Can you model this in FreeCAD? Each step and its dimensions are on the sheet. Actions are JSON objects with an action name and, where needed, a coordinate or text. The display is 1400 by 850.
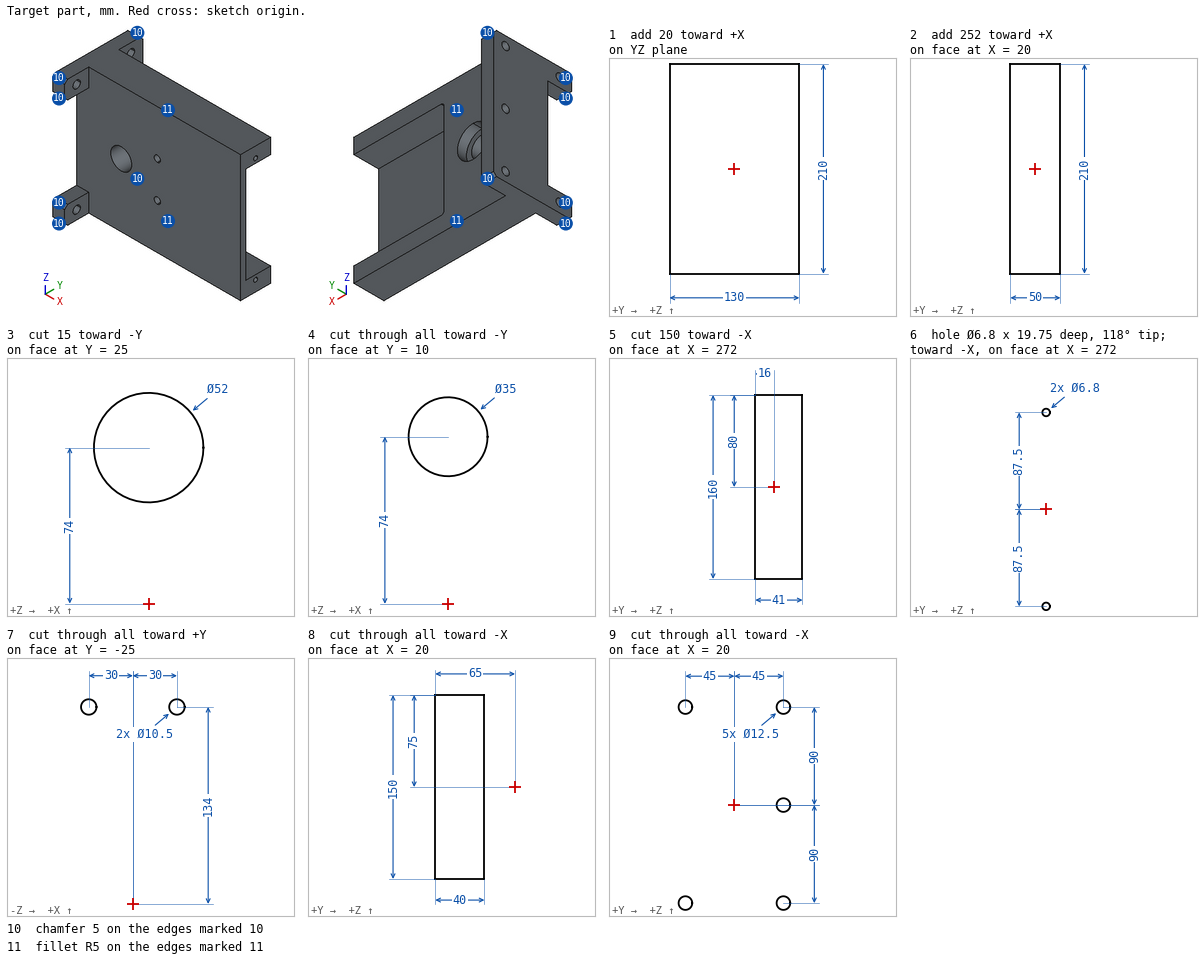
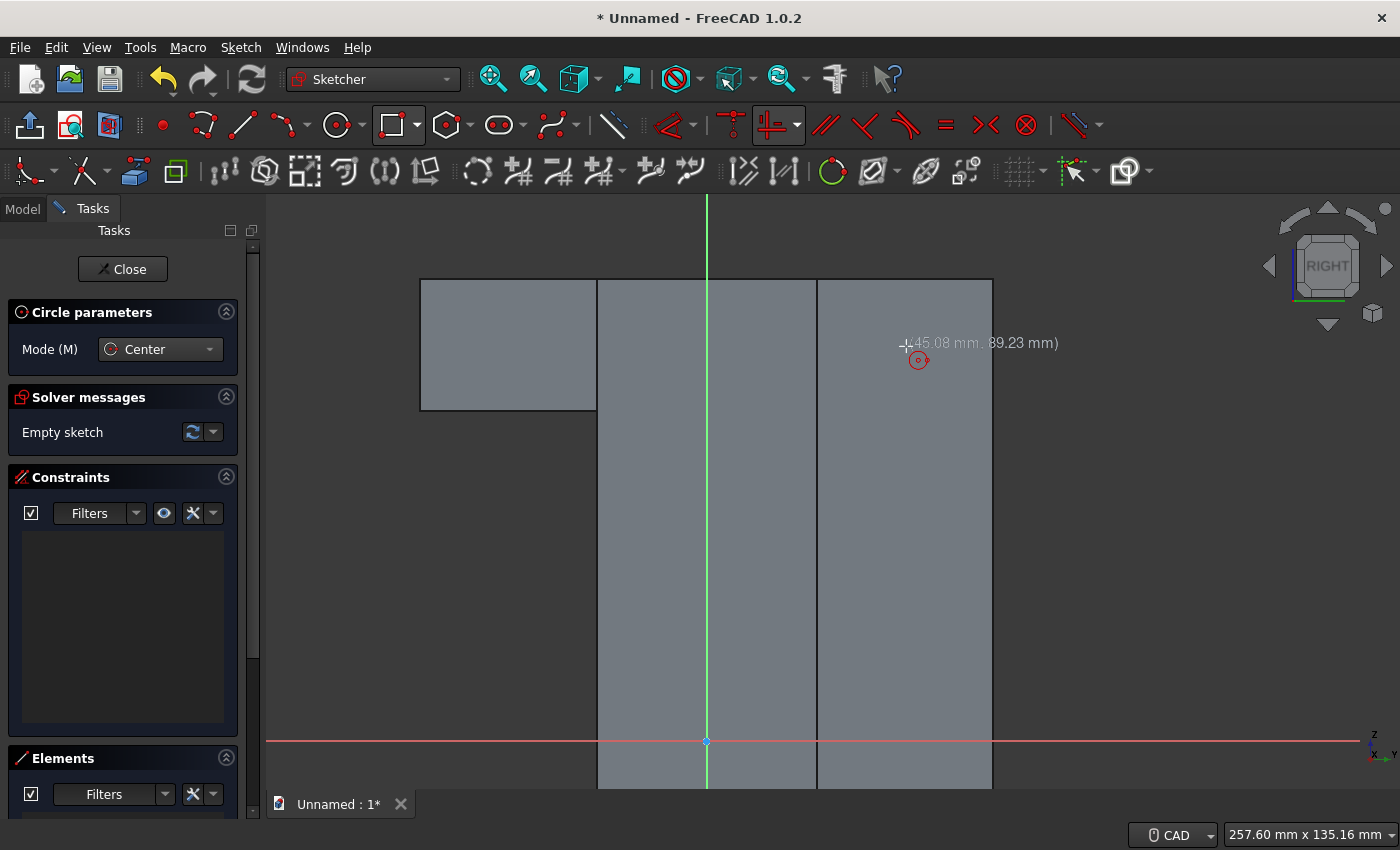
{"action": "left_click", "coordinate": [905, 345]}
{"action": "left_click", "coordinate": [924, 325]}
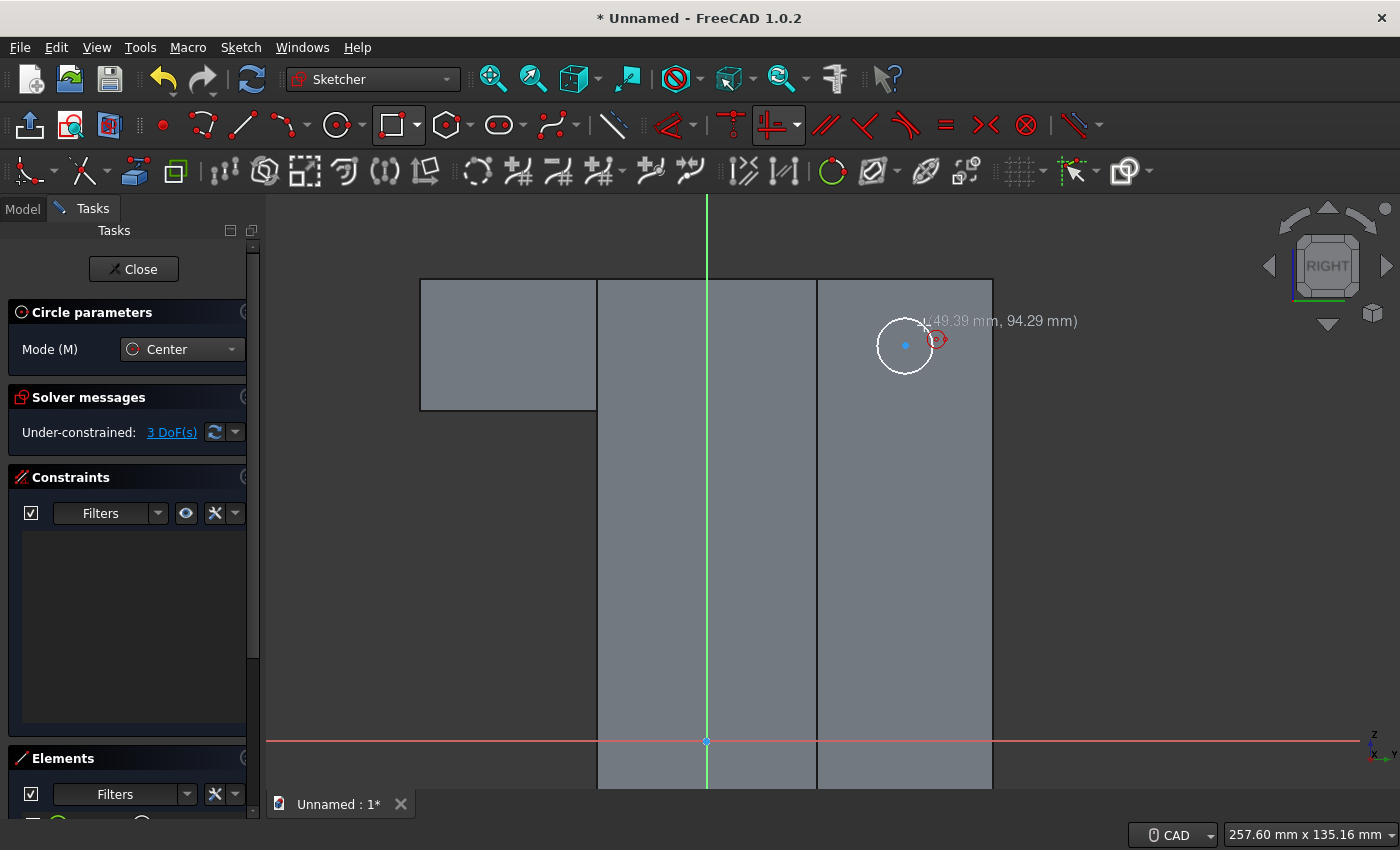
{"action": "left_click", "coordinate": [905, 741]}
{"action": "left_click", "coordinate": [924, 722]}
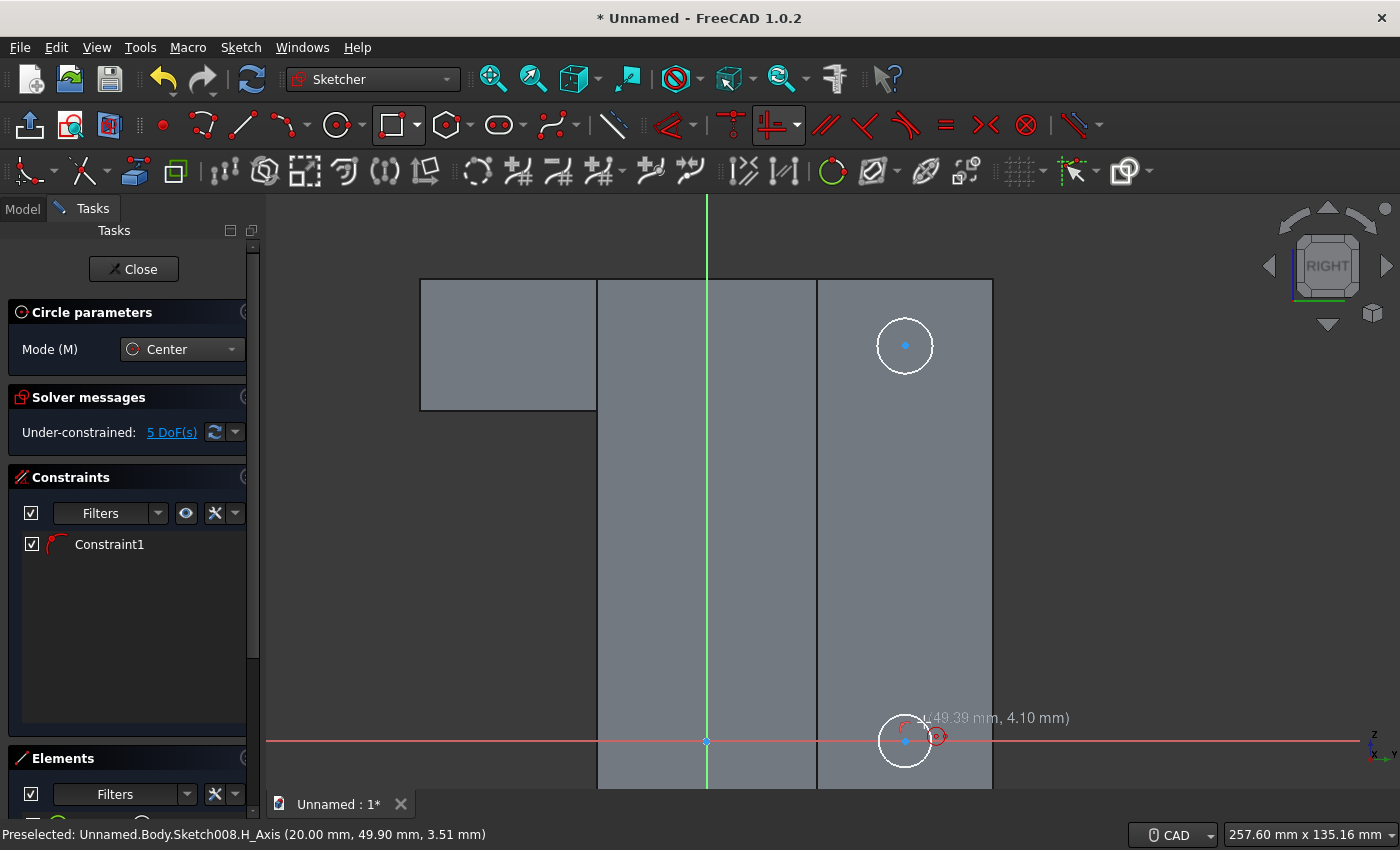
{"action": "scroll", "coordinate": [812, 288], "scroll_direction": "down", "scroll_amount": 4}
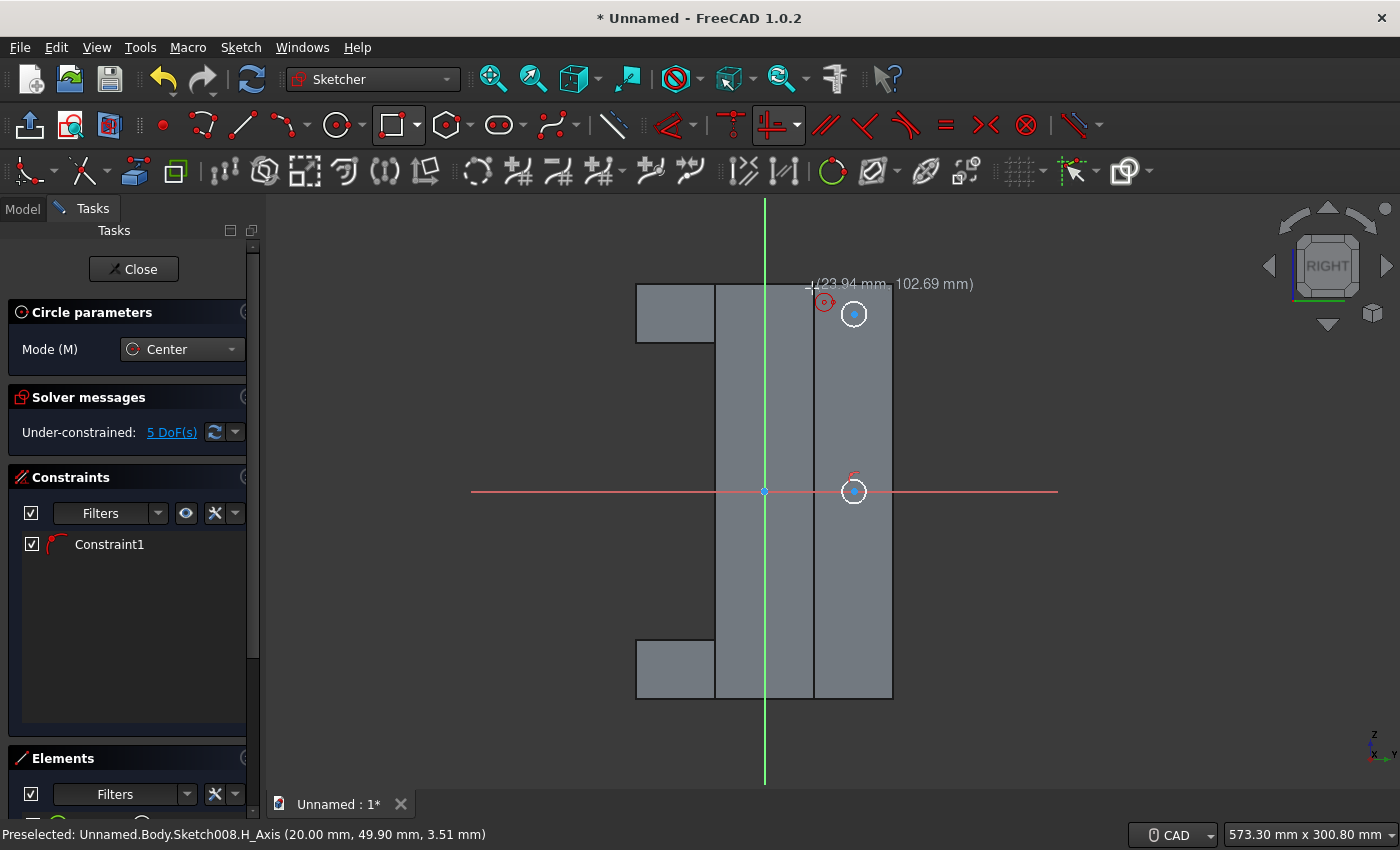
{"action": "scroll", "coordinate": [854, 670], "scroll_direction": "up", "scroll_amount": 4}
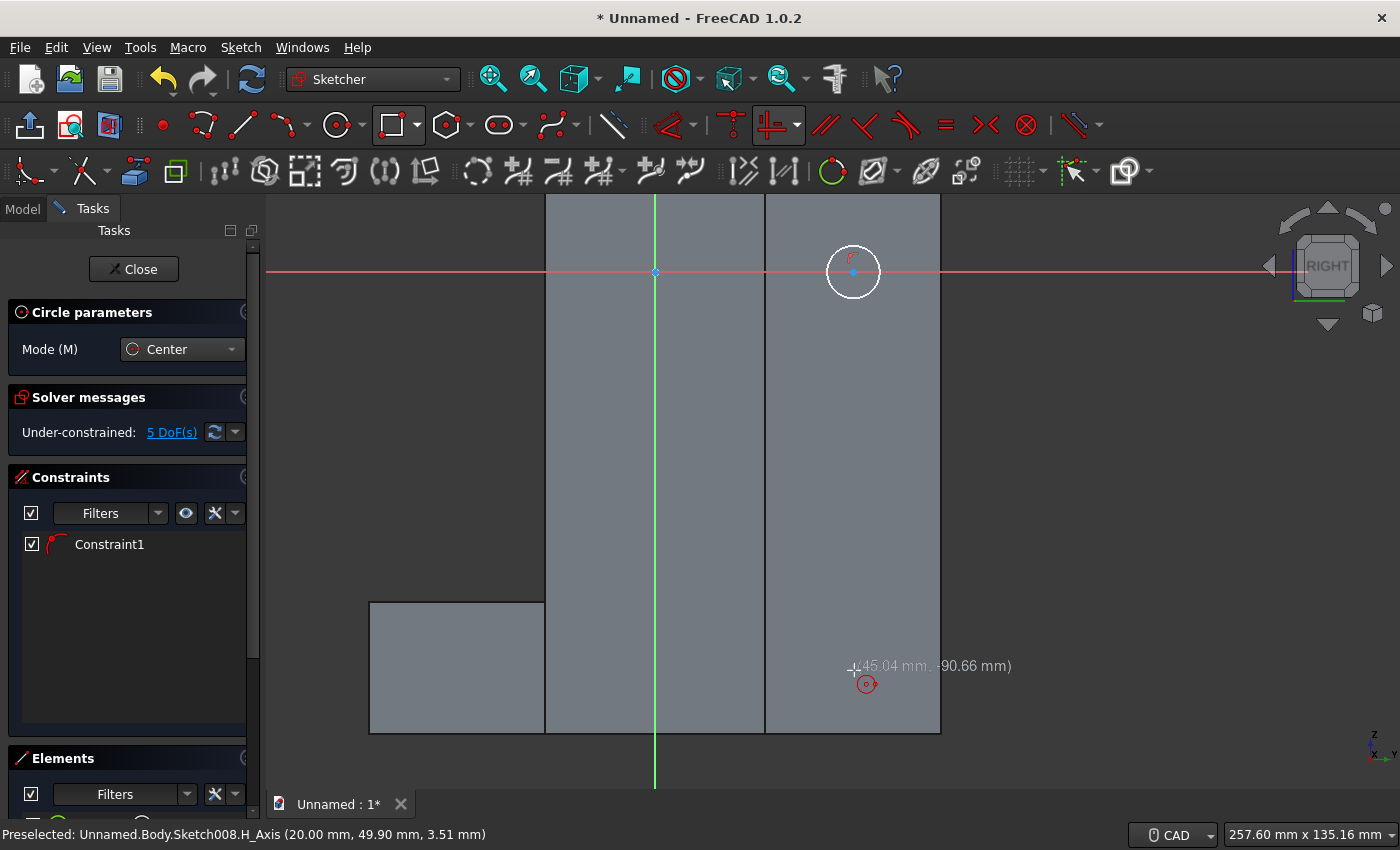
{"action": "left_click", "coordinate": [853, 668]}
{"action": "left_click", "coordinate": [873, 649]}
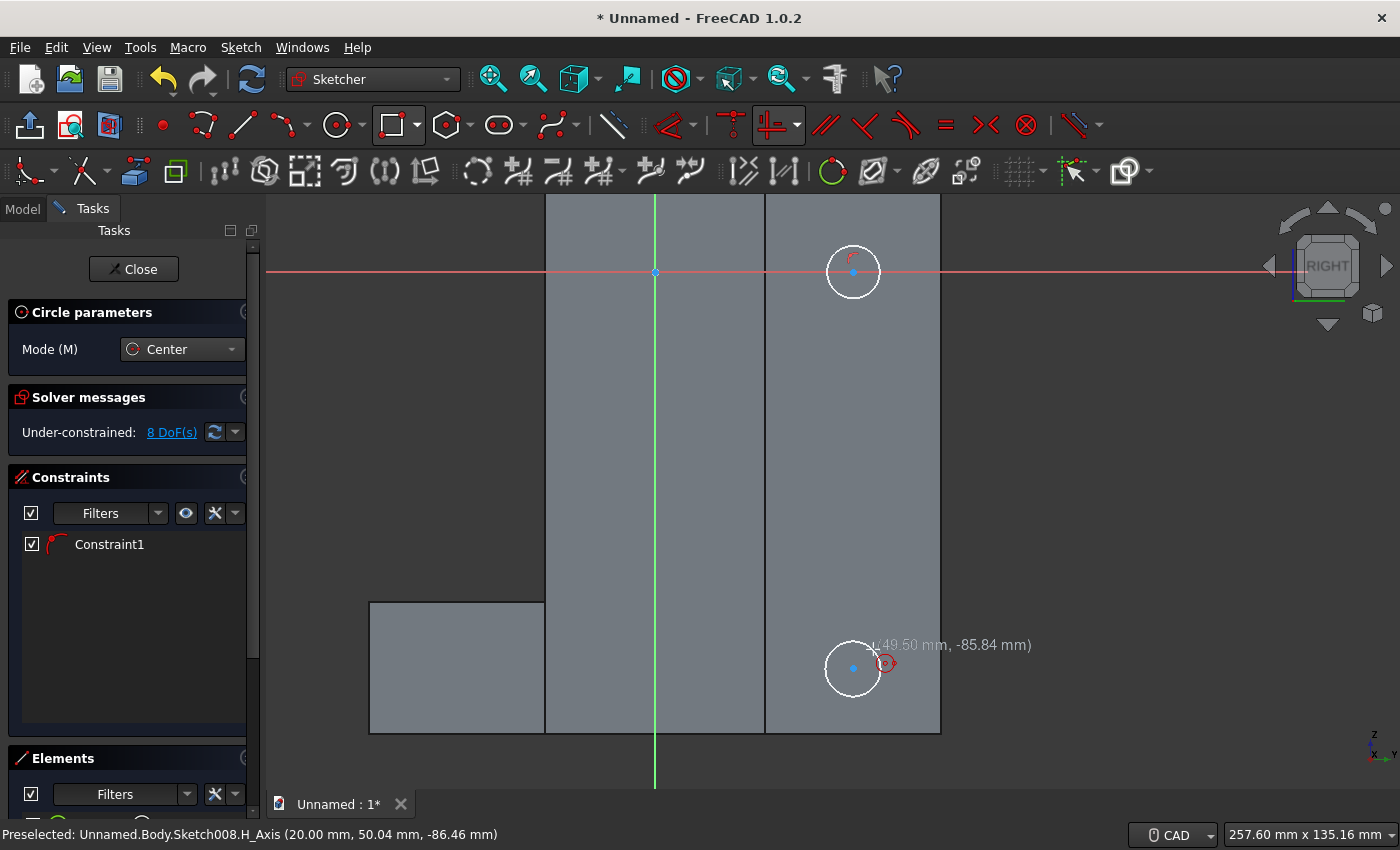
{"action": "scroll", "coordinate": [854, 671], "scroll_direction": "down", "scroll_amount": 4}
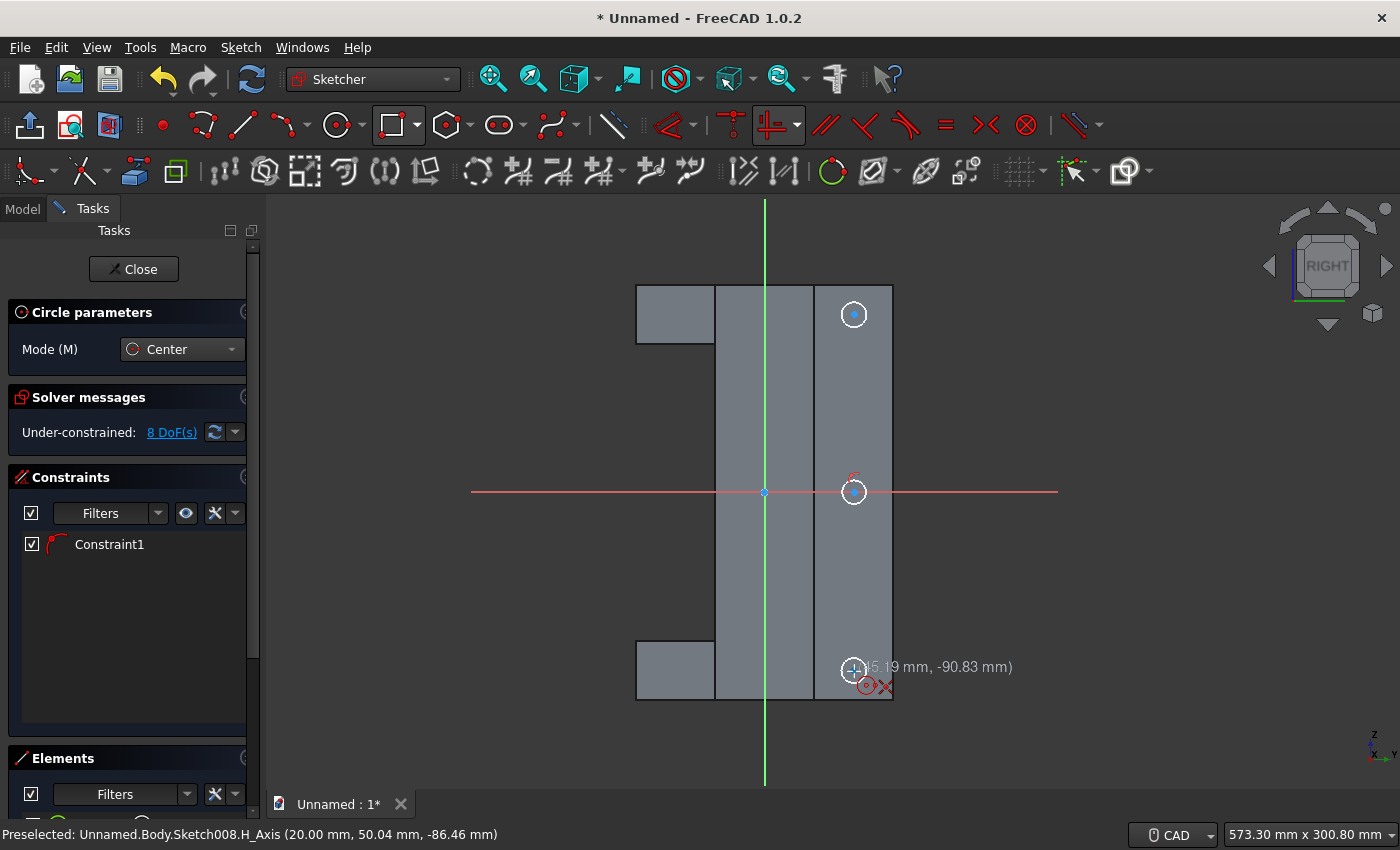
{"action": "scroll", "coordinate": [676, 314], "scroll_direction": "up", "scroll_amount": 4}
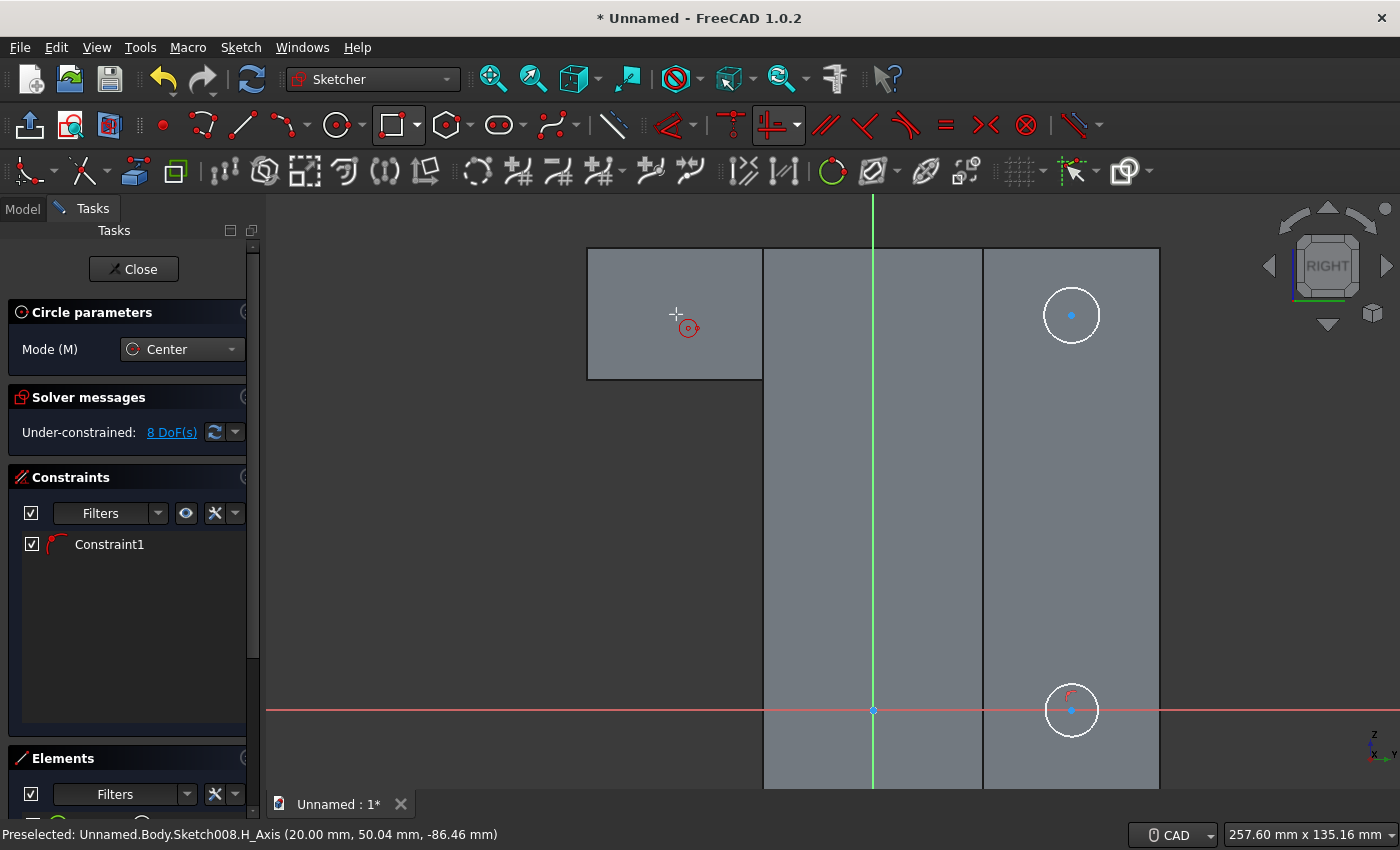
{"action": "left_click", "coordinate": [675, 314]}
{"action": "left_click", "coordinate": [695, 295]}